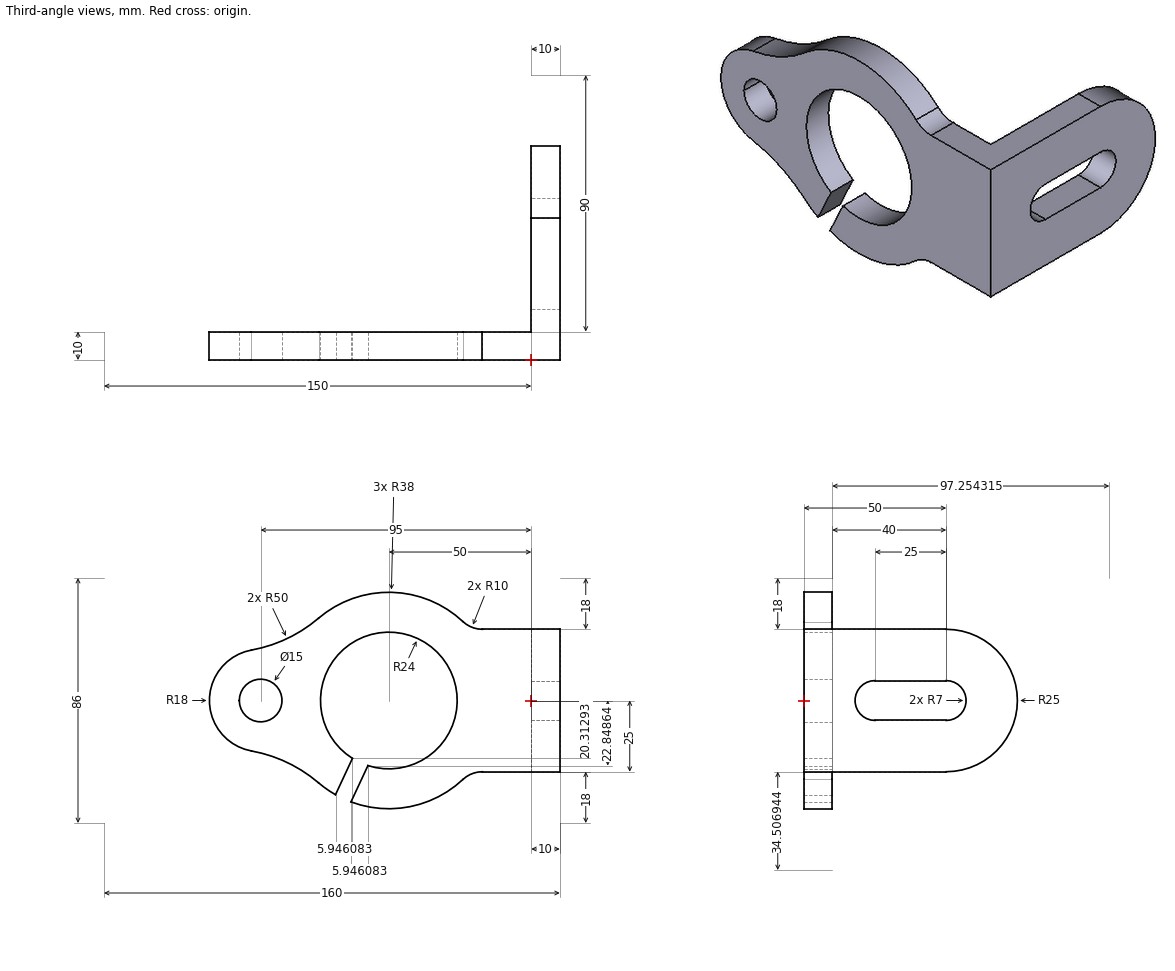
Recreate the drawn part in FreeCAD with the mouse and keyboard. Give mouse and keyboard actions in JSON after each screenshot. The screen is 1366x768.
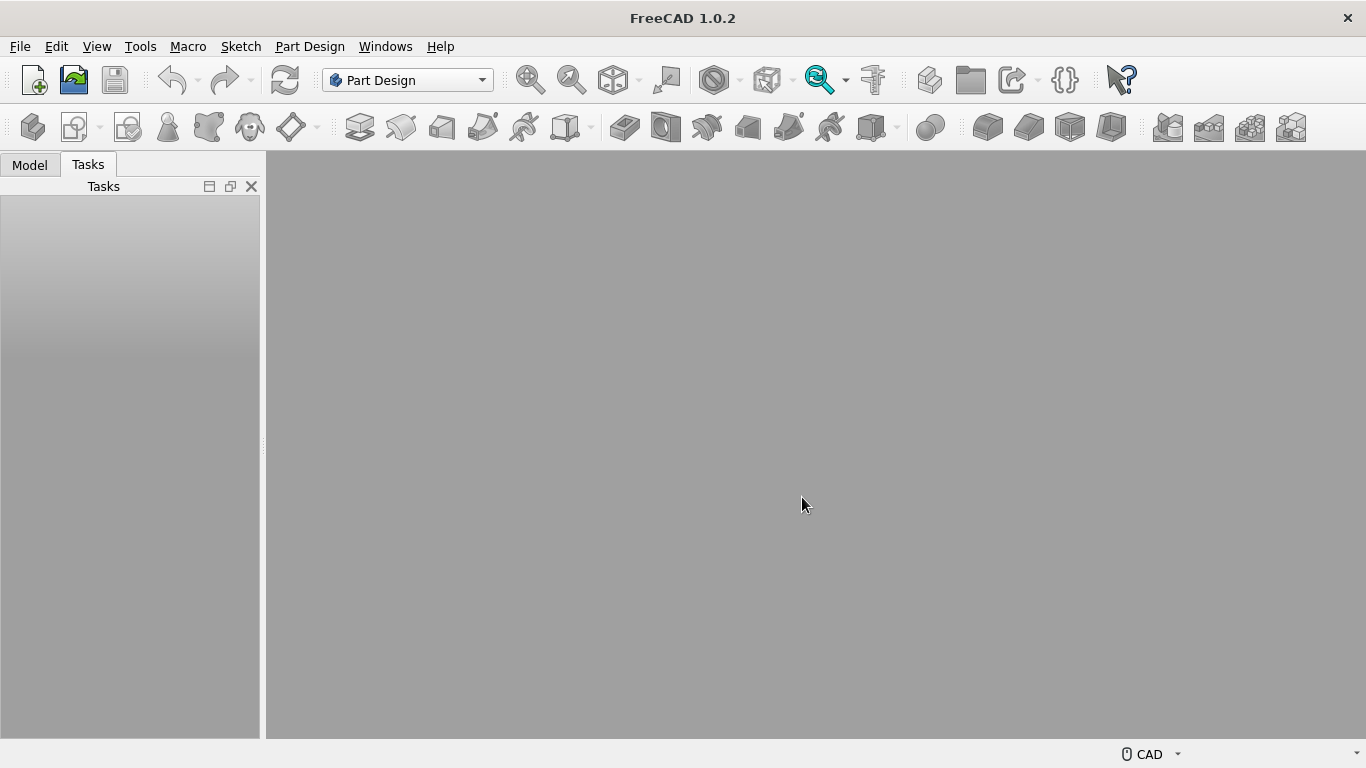
{"action": "left_click", "coordinate": [33, 80]}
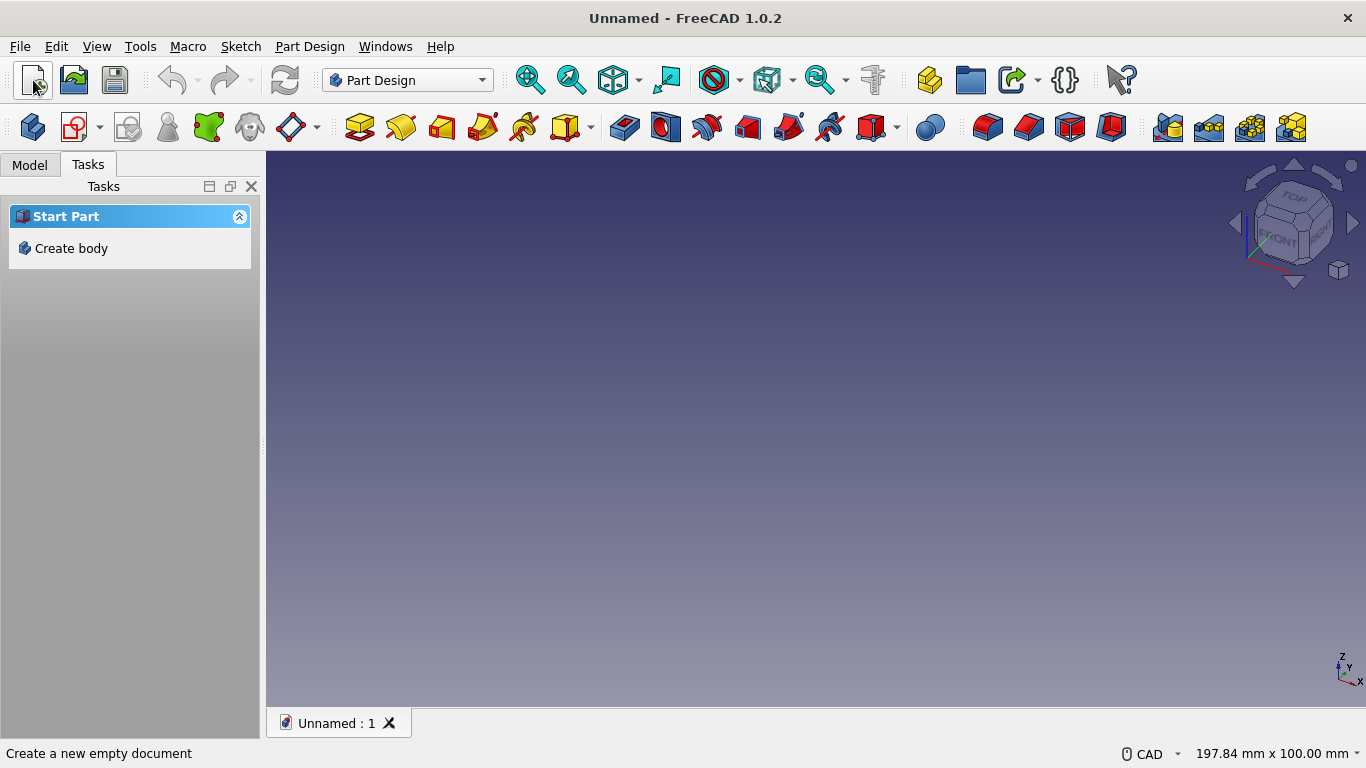
{"action": "left_click", "coordinate": [74, 128]}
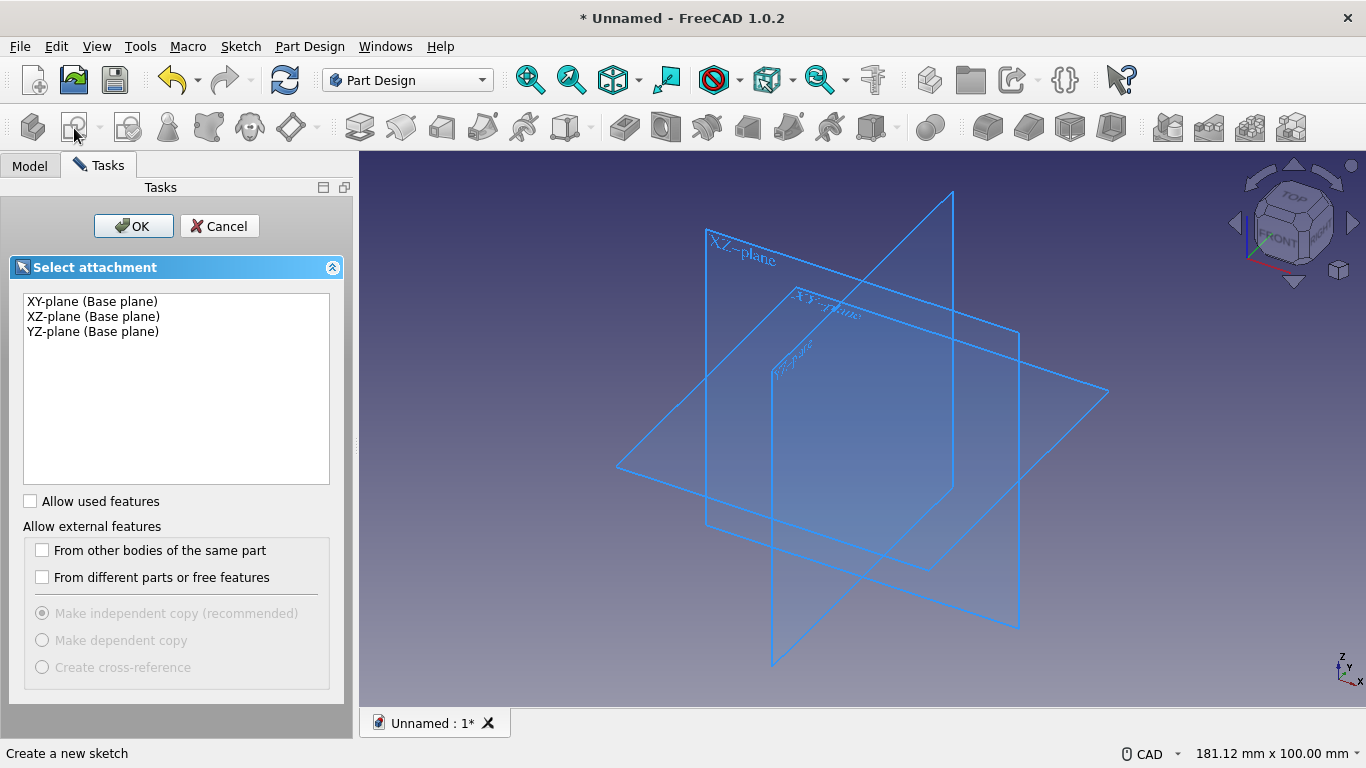
{"action": "left_click", "coordinate": [84, 302]}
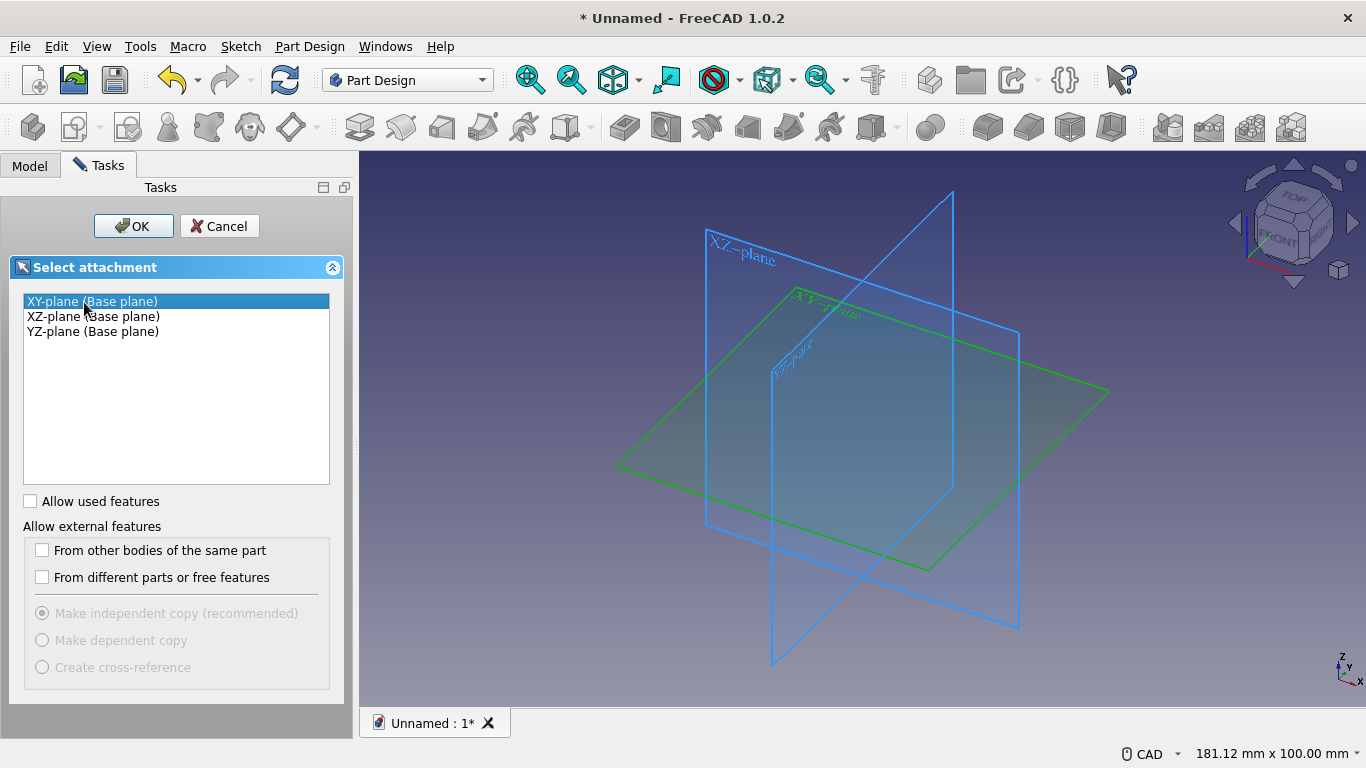
{"action": "left_click", "coordinate": [134, 226]}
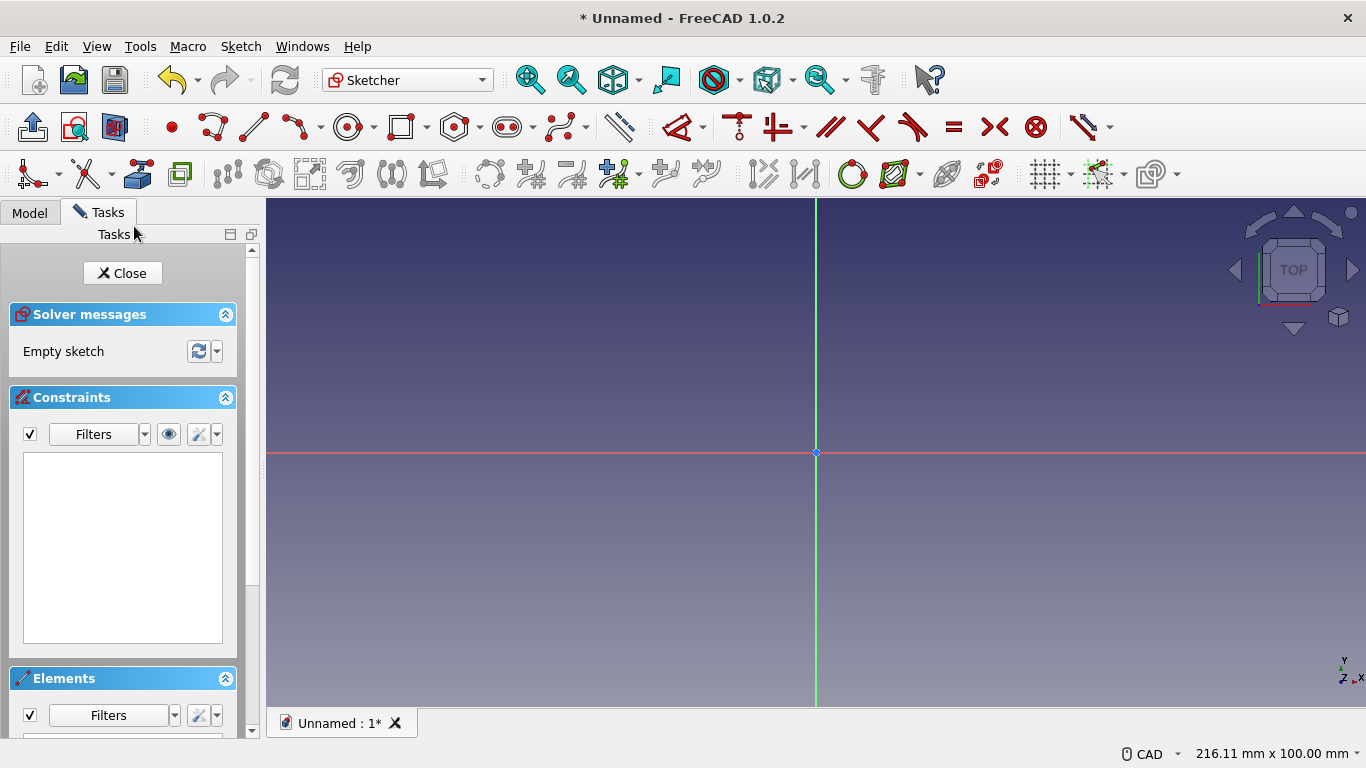
{"action": "scroll", "coordinate": [1098, 679], "scroll_direction": "down", "scroll_amount": 3}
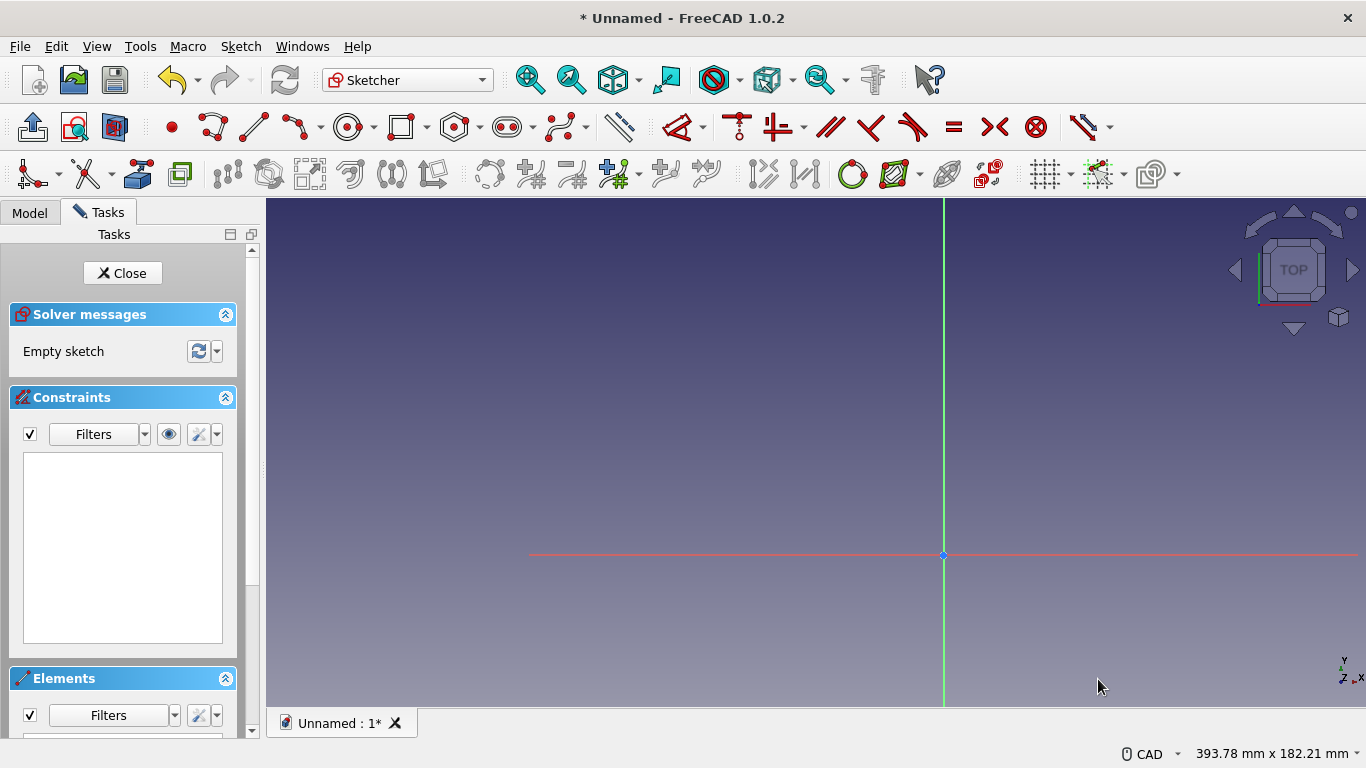
{"action": "key", "text": "g m"}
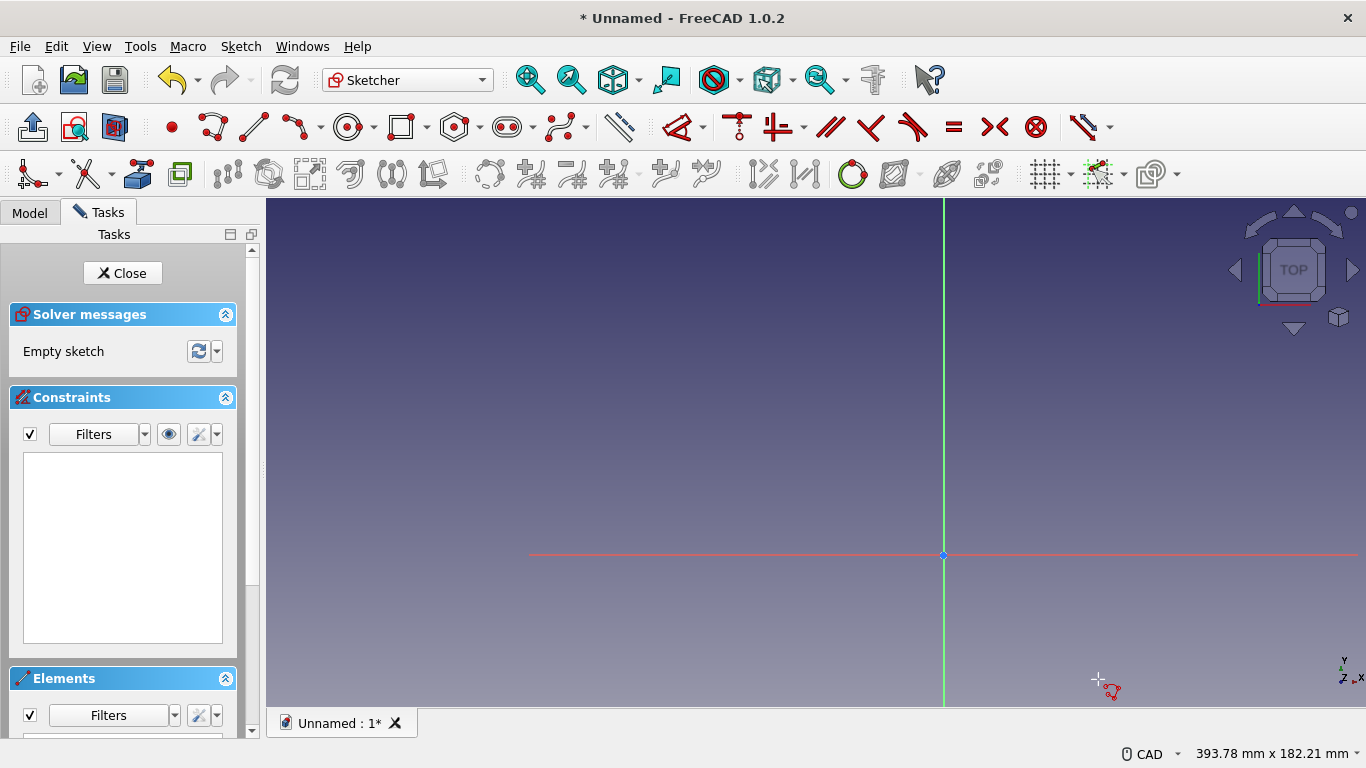
{"action": "left_click", "coordinate": [972, 555]}
{"action": "left_click", "coordinate": [972, 276]}
{"action": "left_click", "coordinate": [944, 276]}
{"action": "left_click", "coordinate": [935, 527]}
{"action": "left_click", "coordinate": [525, 527]}
{"action": "left_click", "coordinate": [525, 546]}
{"action": "left_click", "coordinate": [972, 555]}
{"action": "key", "text": "Escape"}
{"action": "key", "text": "Escape"}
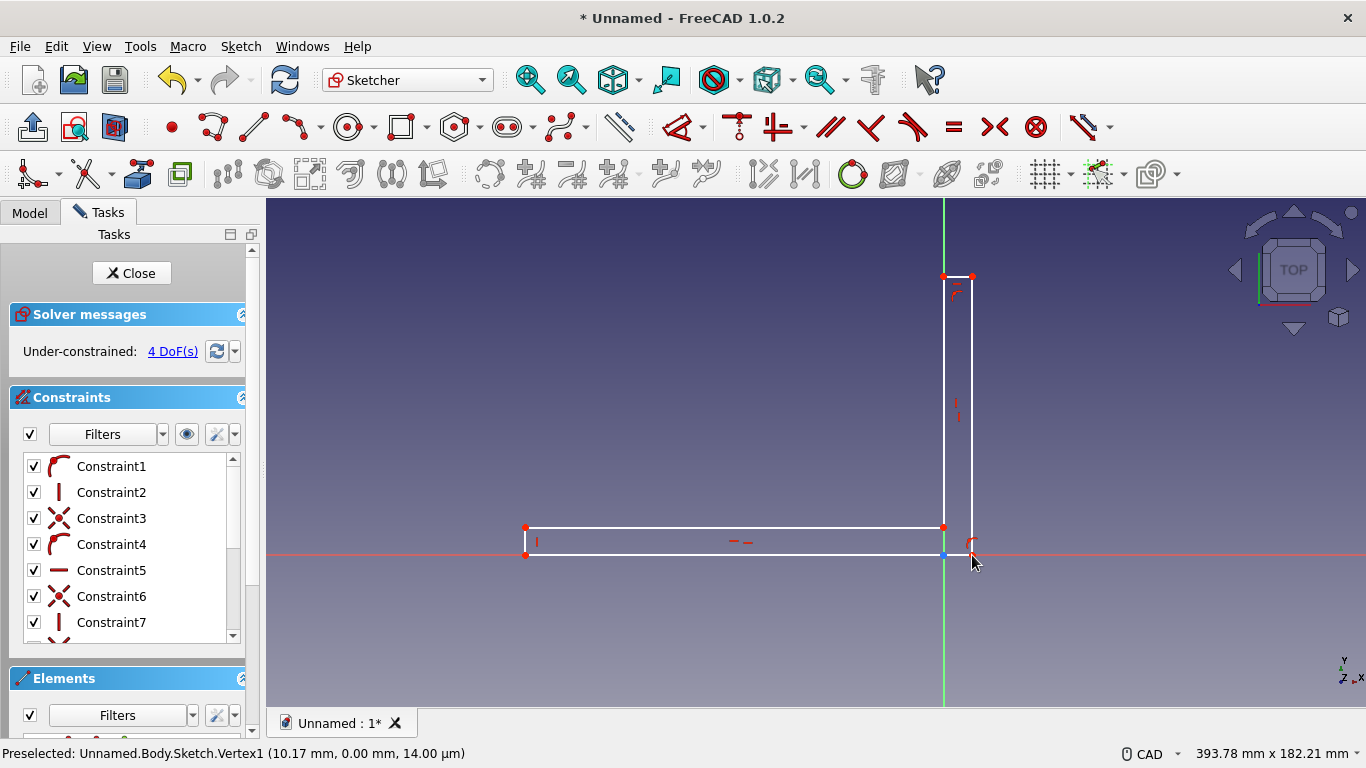
{"action": "scroll", "coordinate": [961, 277], "scroll_direction": "up", "scroll_amount": 2}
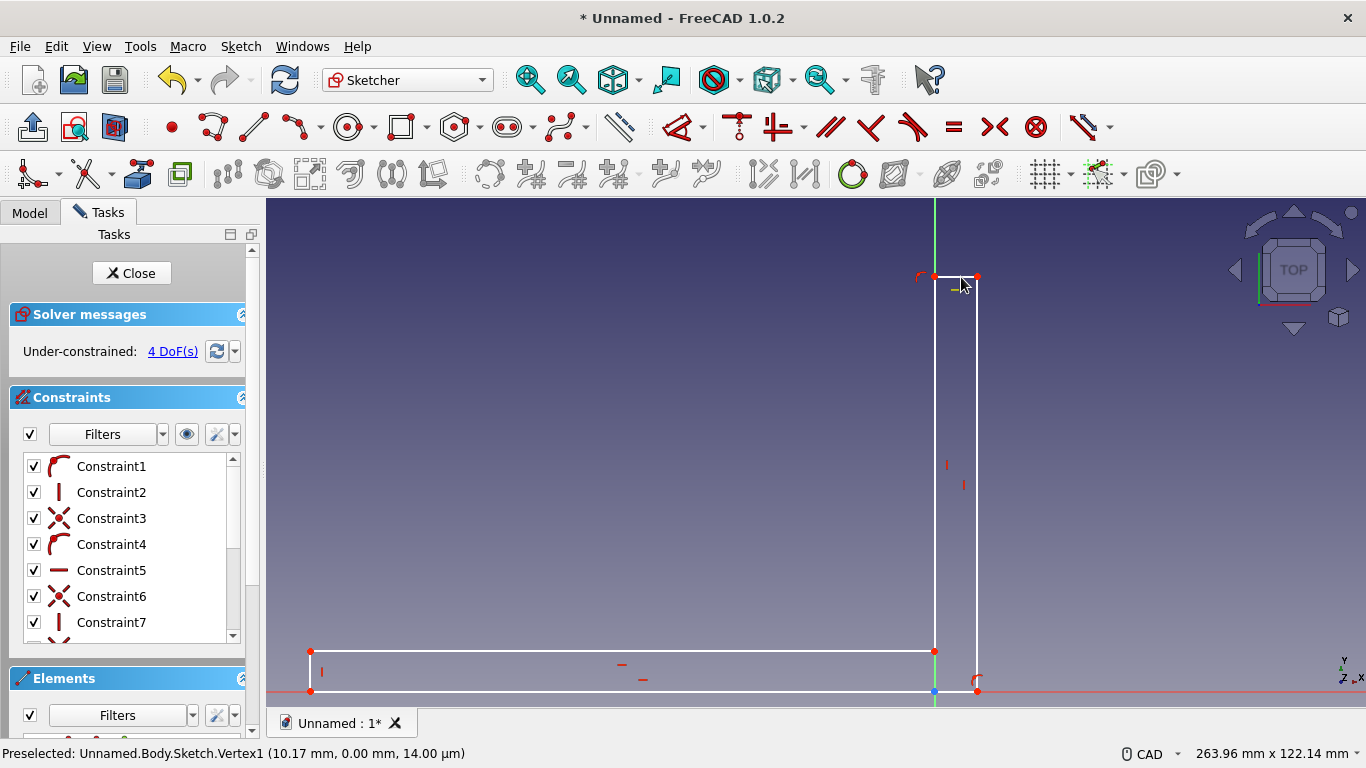
{"action": "left_click", "coordinate": [960, 277]}